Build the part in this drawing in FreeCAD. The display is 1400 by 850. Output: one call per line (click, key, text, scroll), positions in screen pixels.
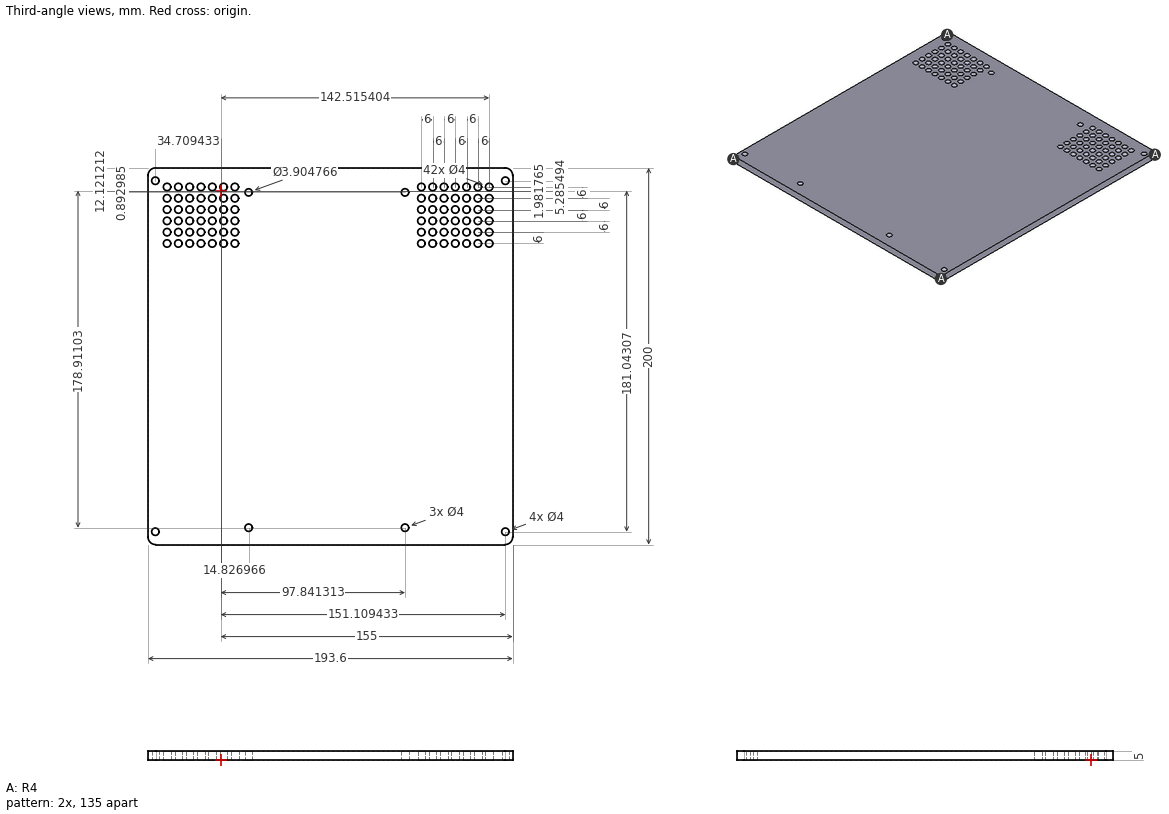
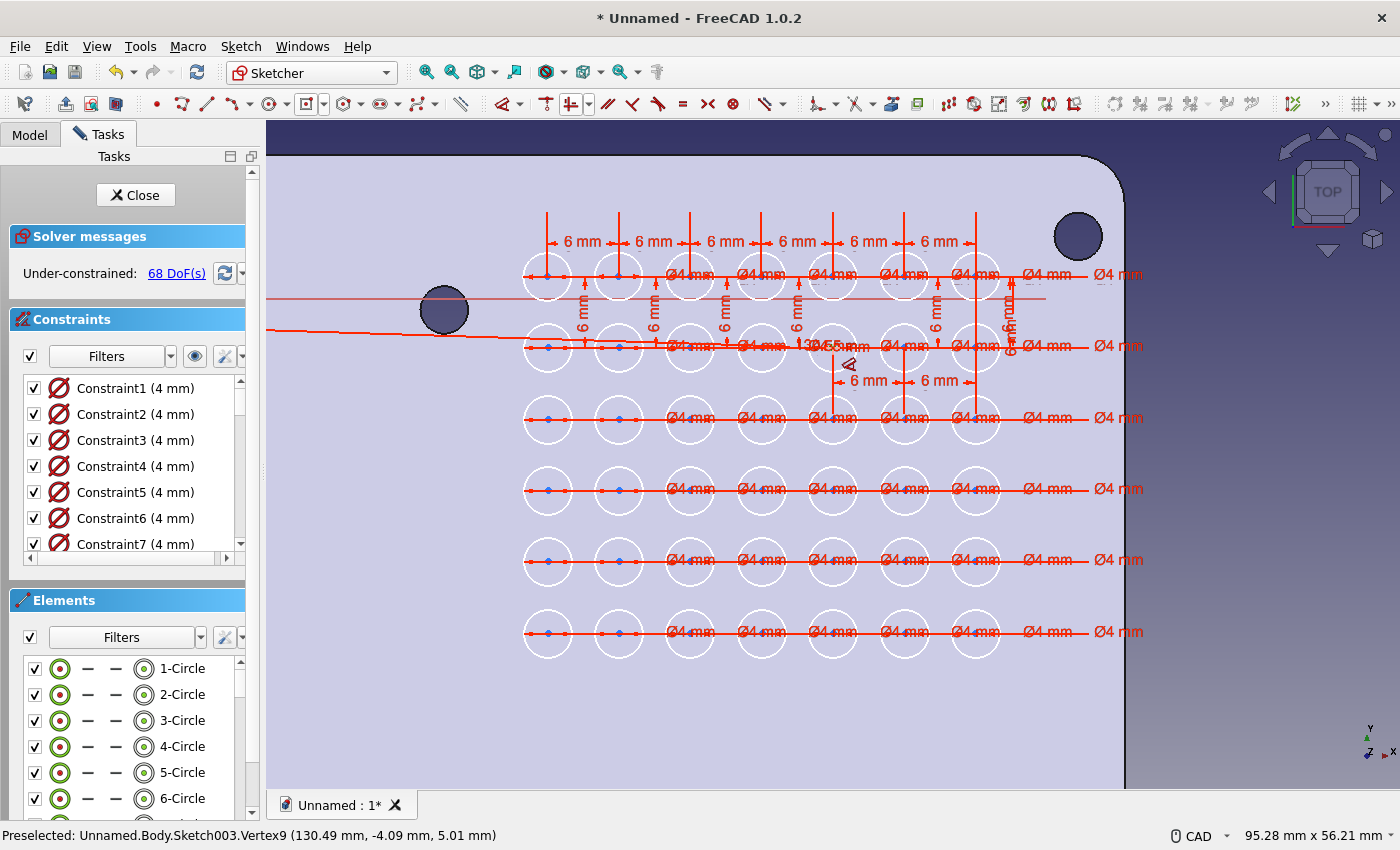
click(762, 348)
click(797, 382)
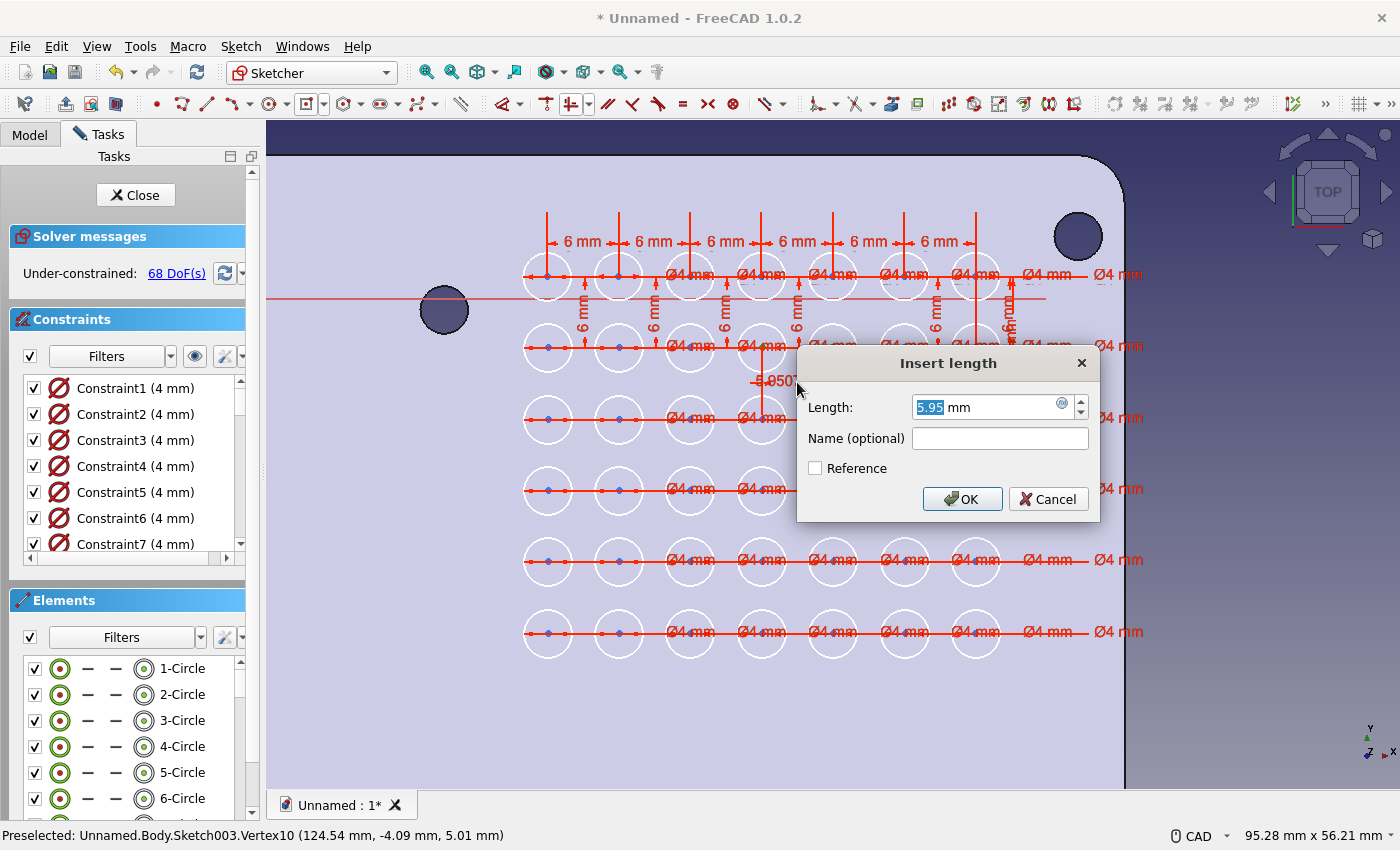
text(6)
key(Return)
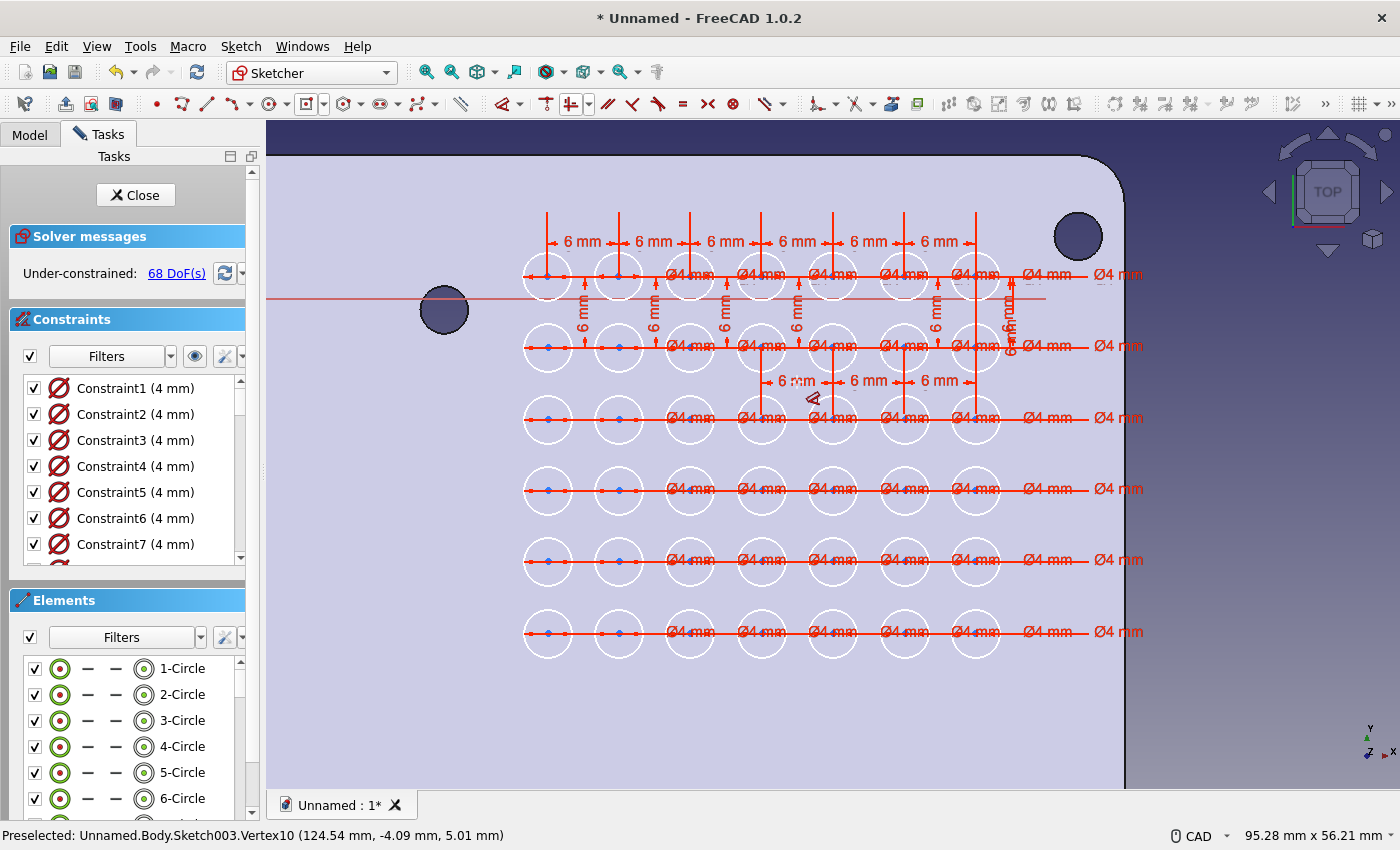
click(761, 277)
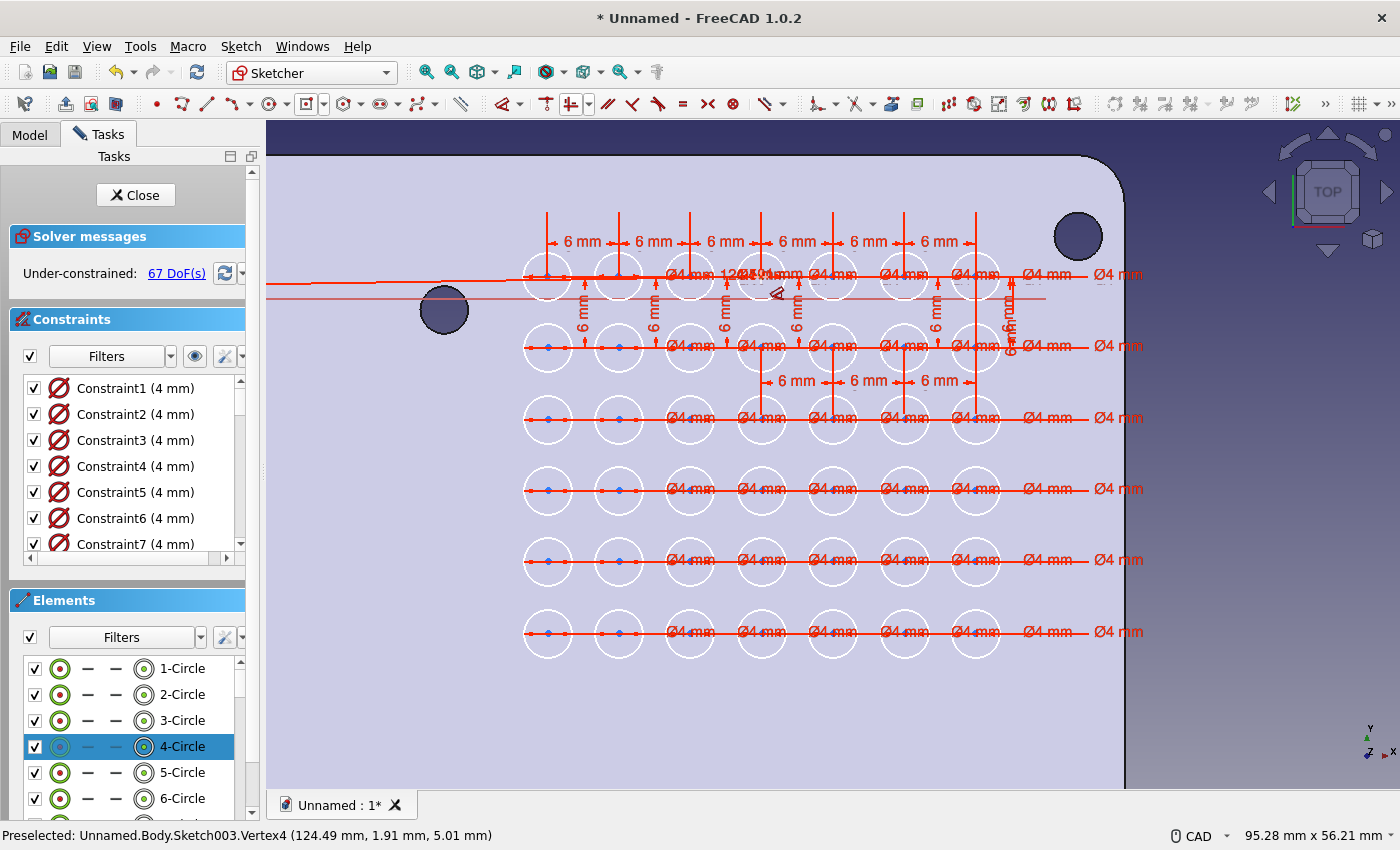
click(761, 348)
click(727, 329)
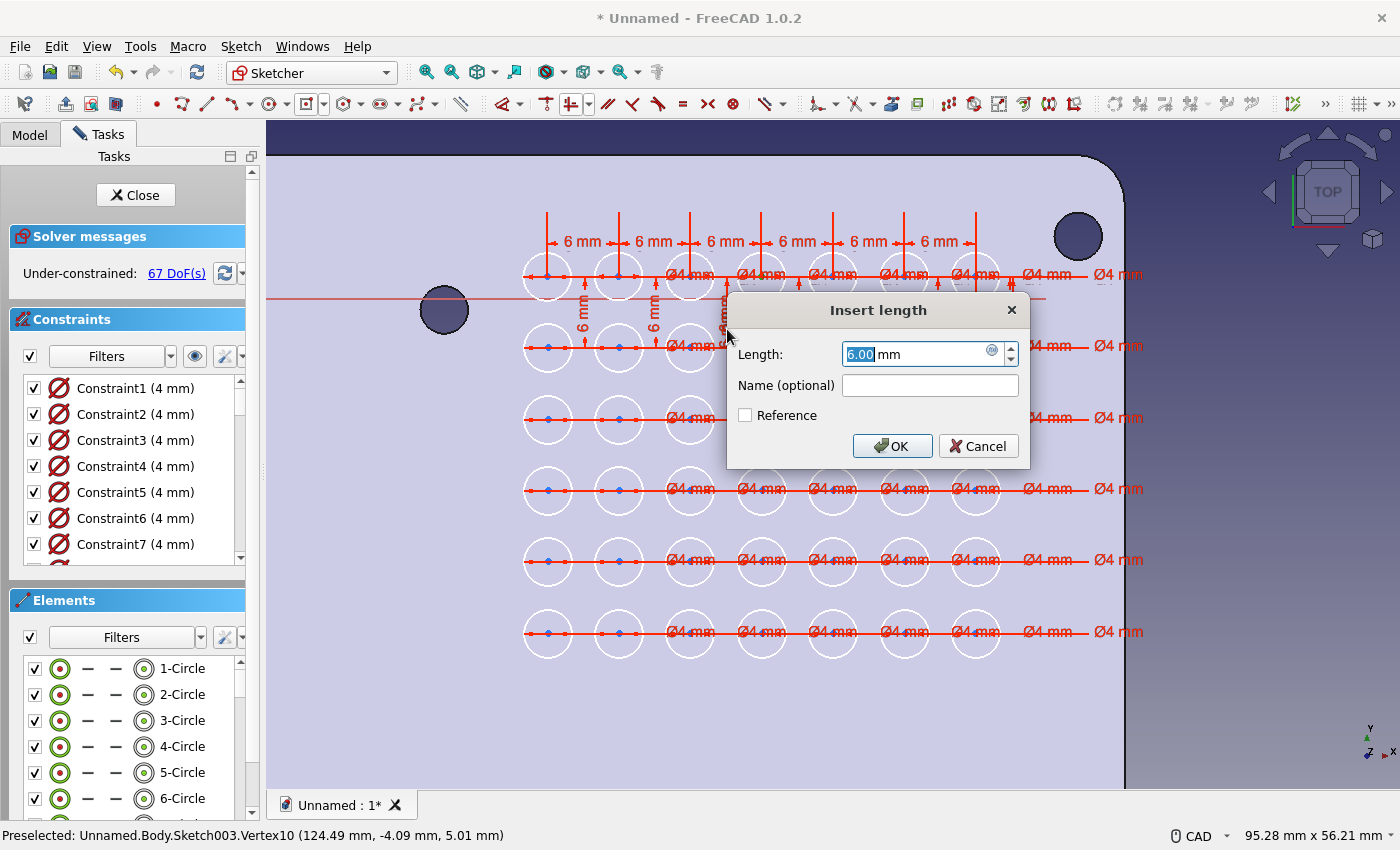
text(6)
key(Return)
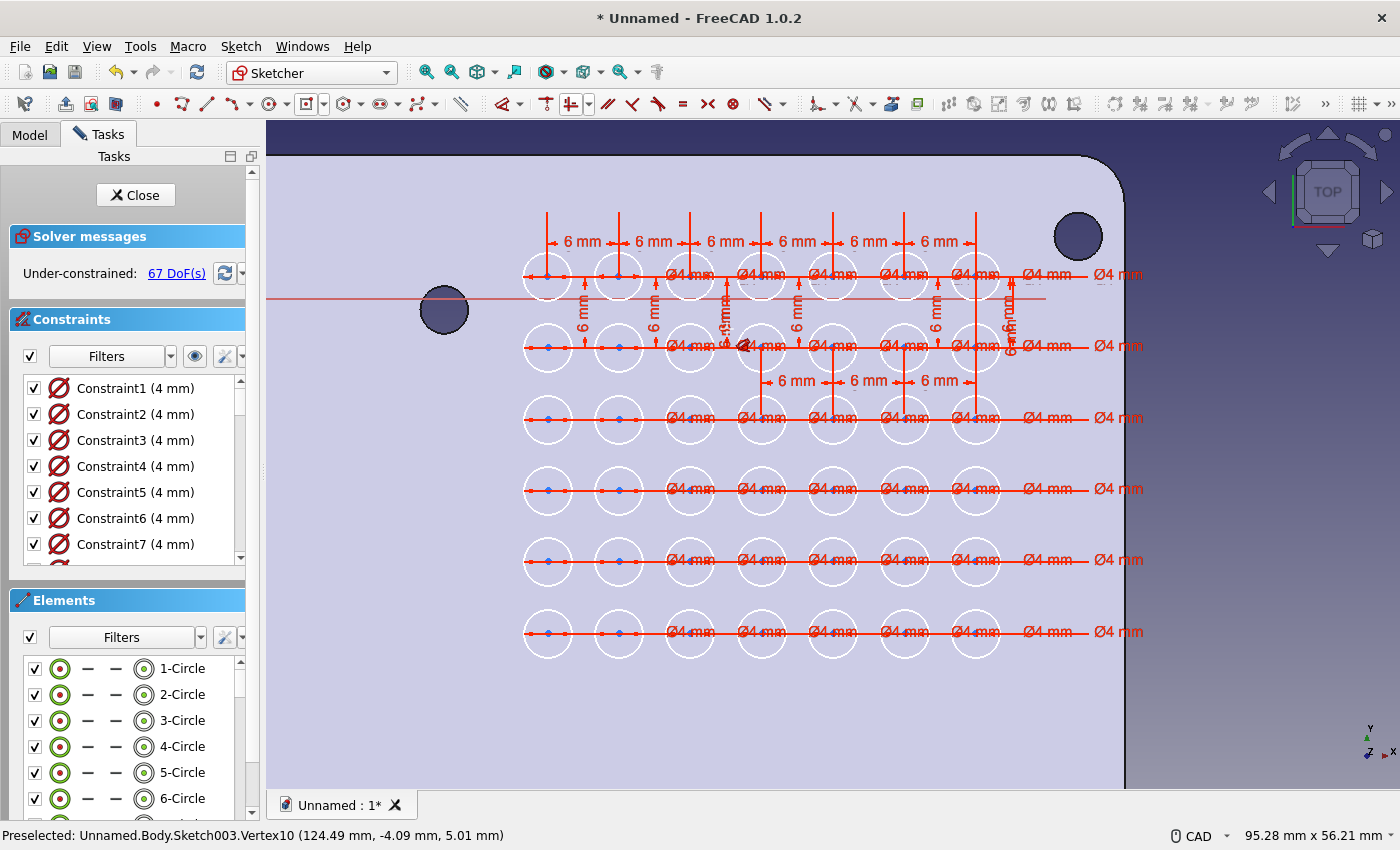
click(761, 348)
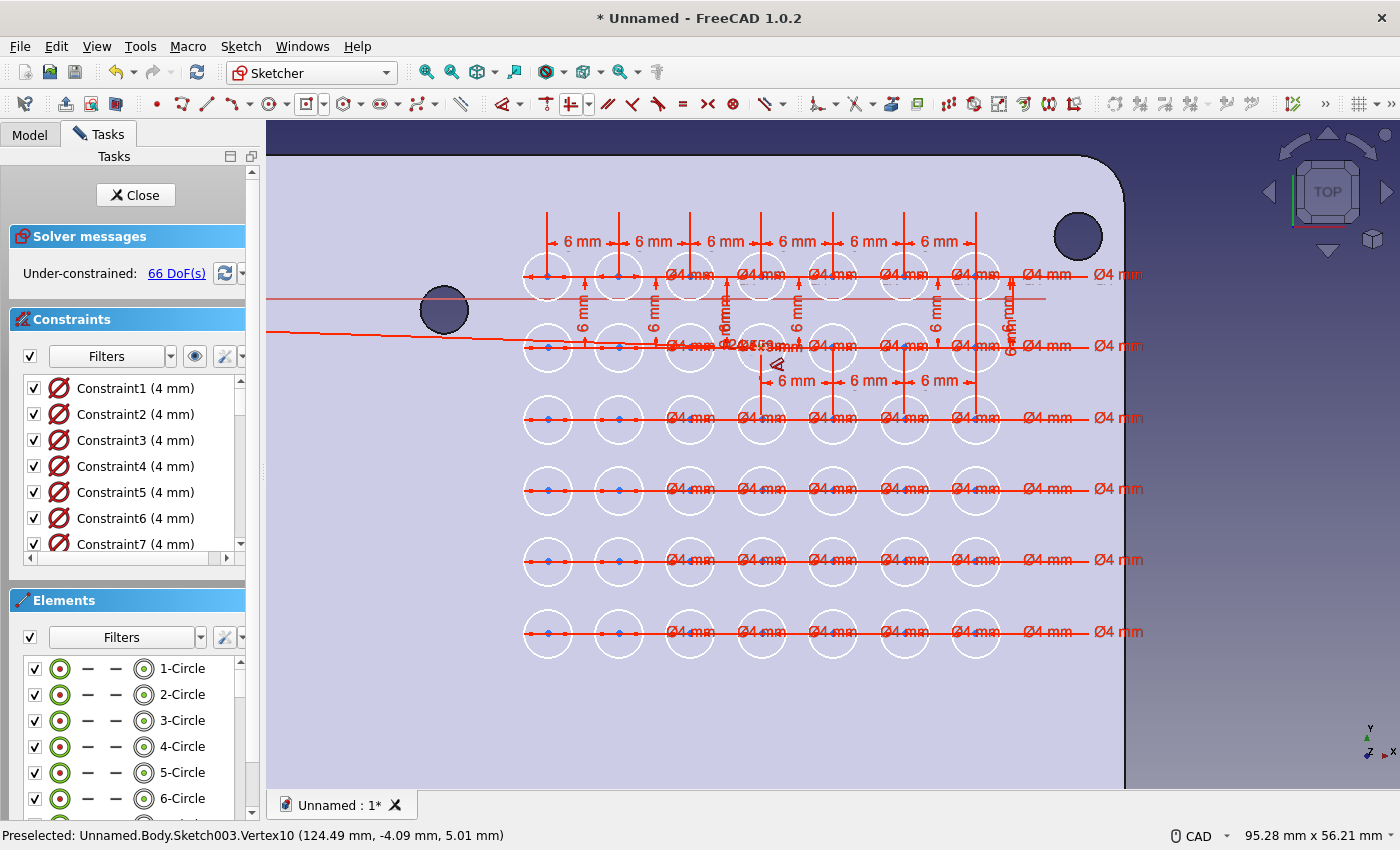
click(690, 348)
click(726, 382)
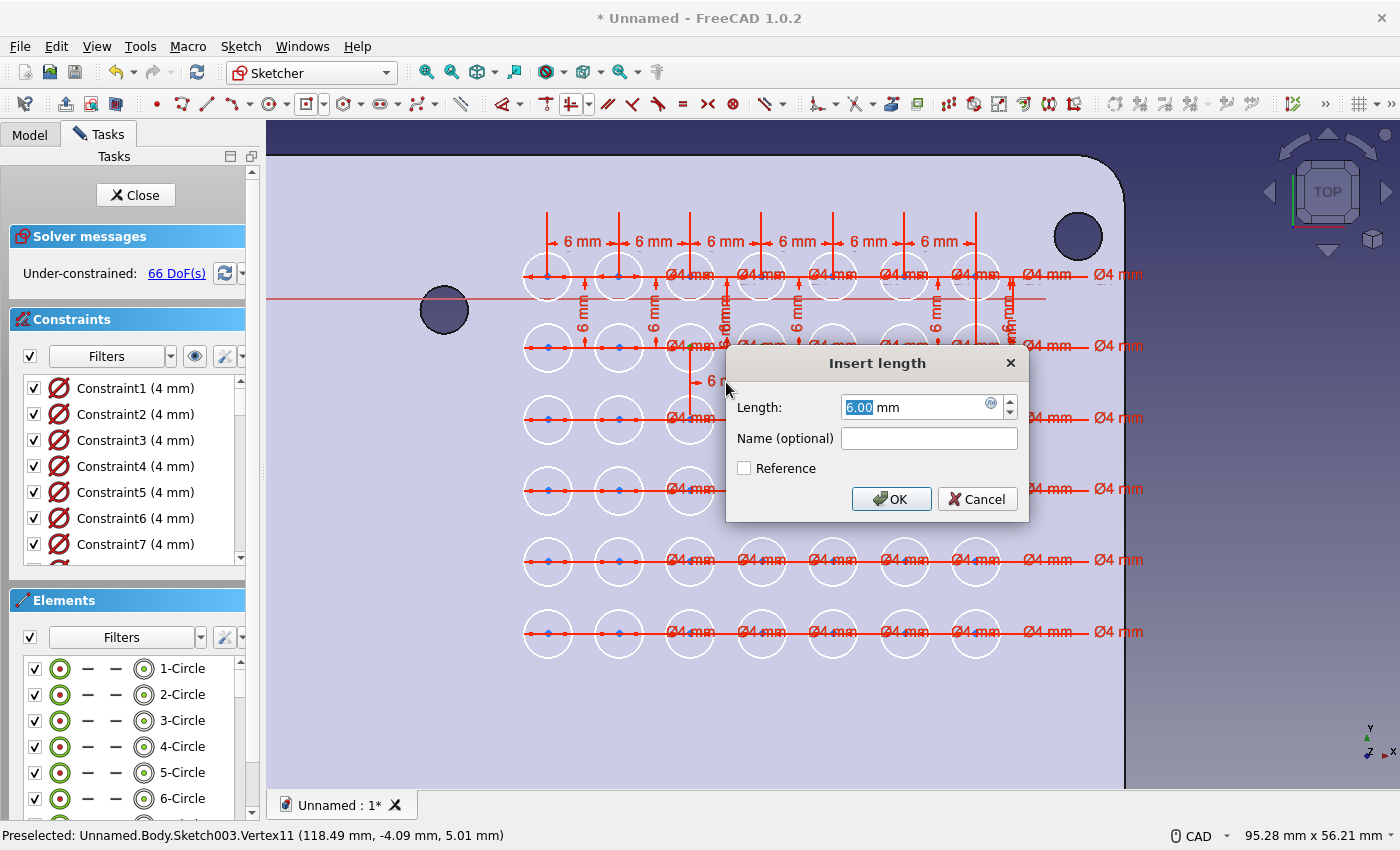
text(6)
key(Return)